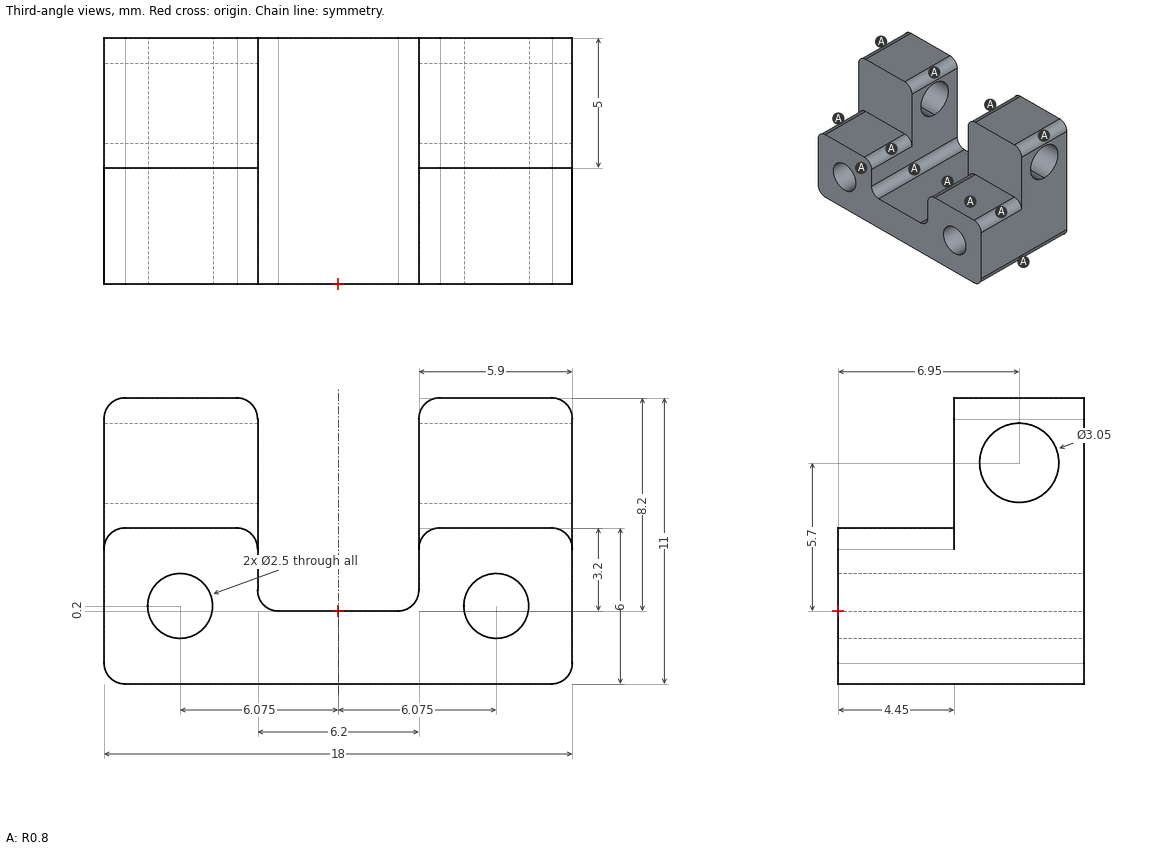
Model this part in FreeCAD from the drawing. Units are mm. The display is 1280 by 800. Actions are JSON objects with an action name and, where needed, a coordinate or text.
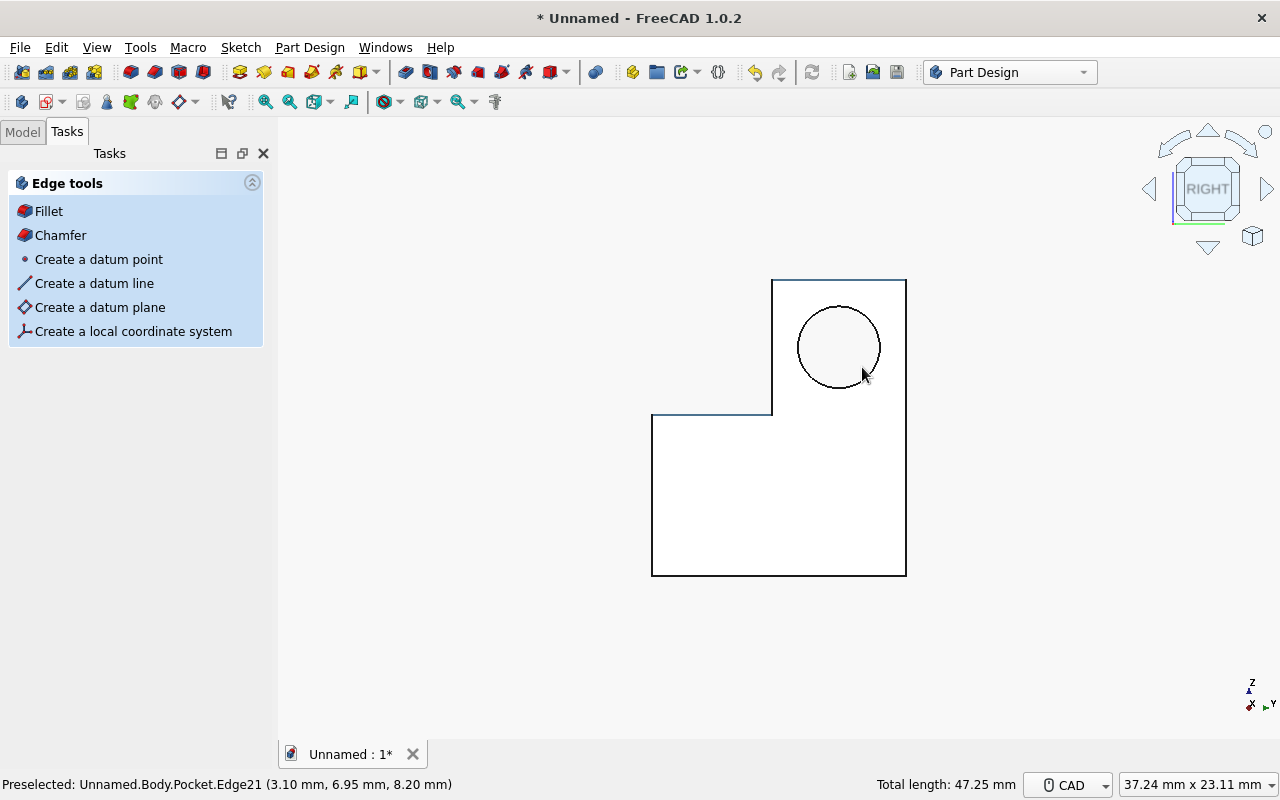
{"action": "left_click", "coordinate": [779, 575], "text": "ctrl"}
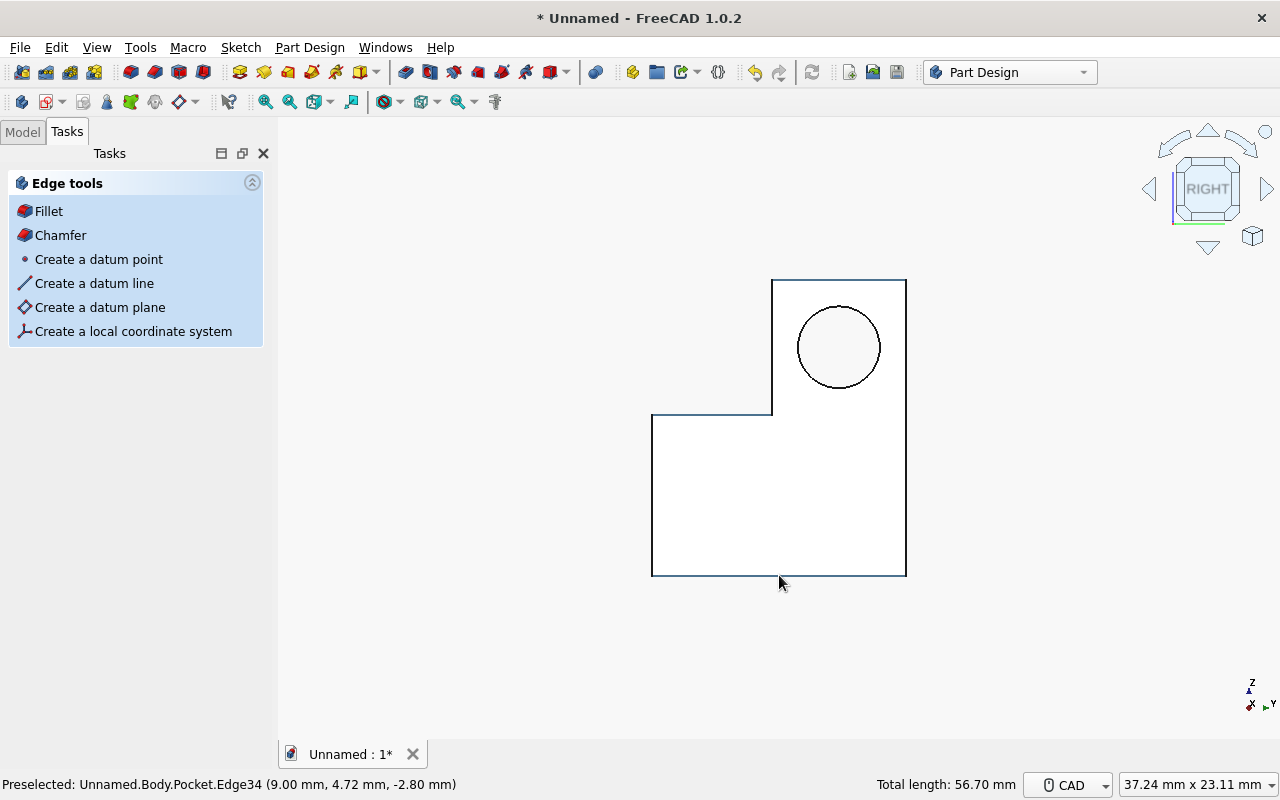
{"action": "key", "text": "5"}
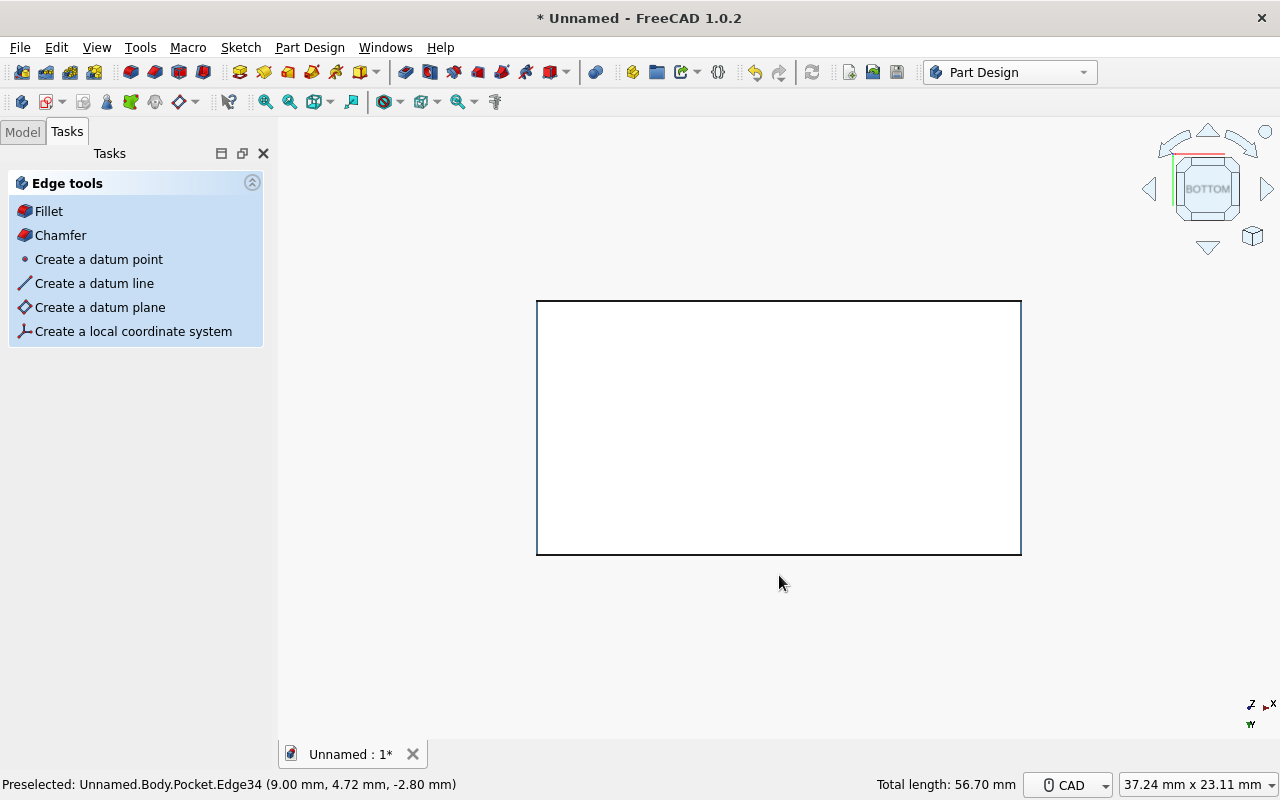
{"action": "key", "text": "4"}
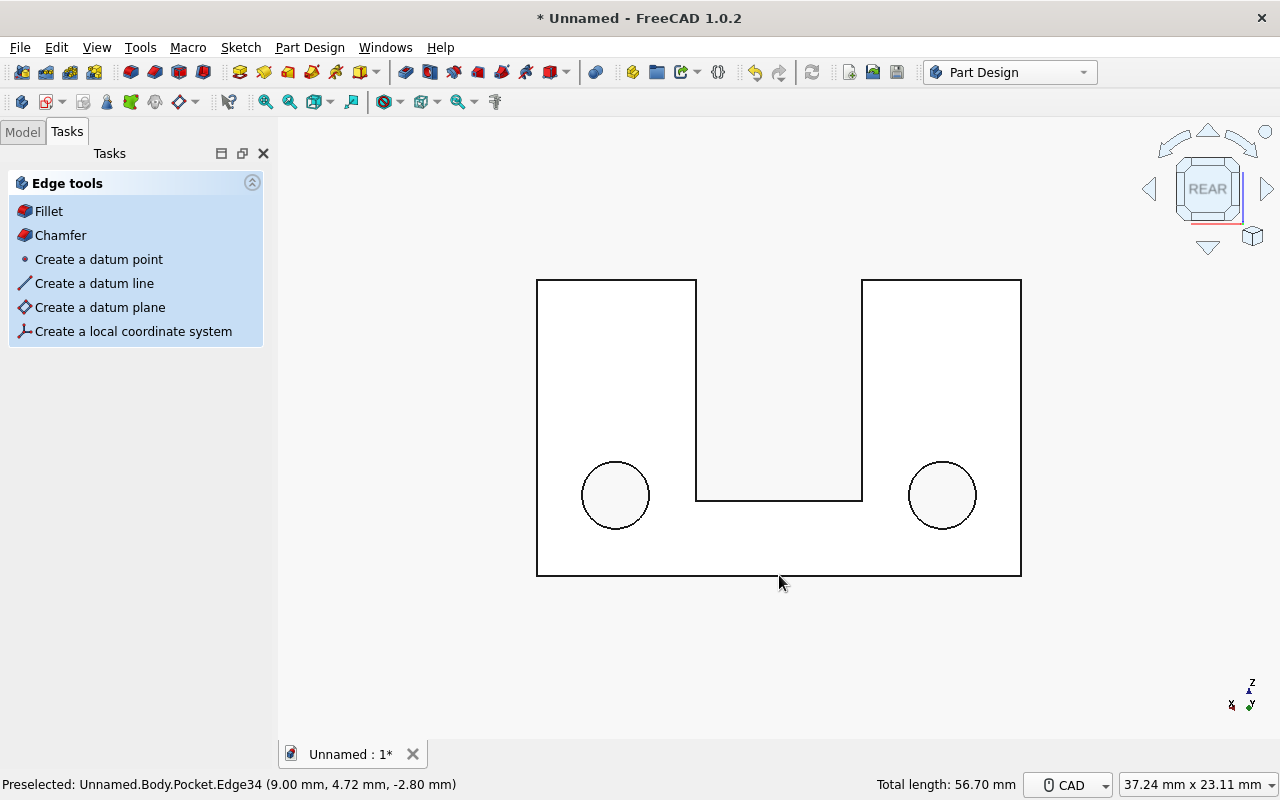
{"action": "key", "text": "6"}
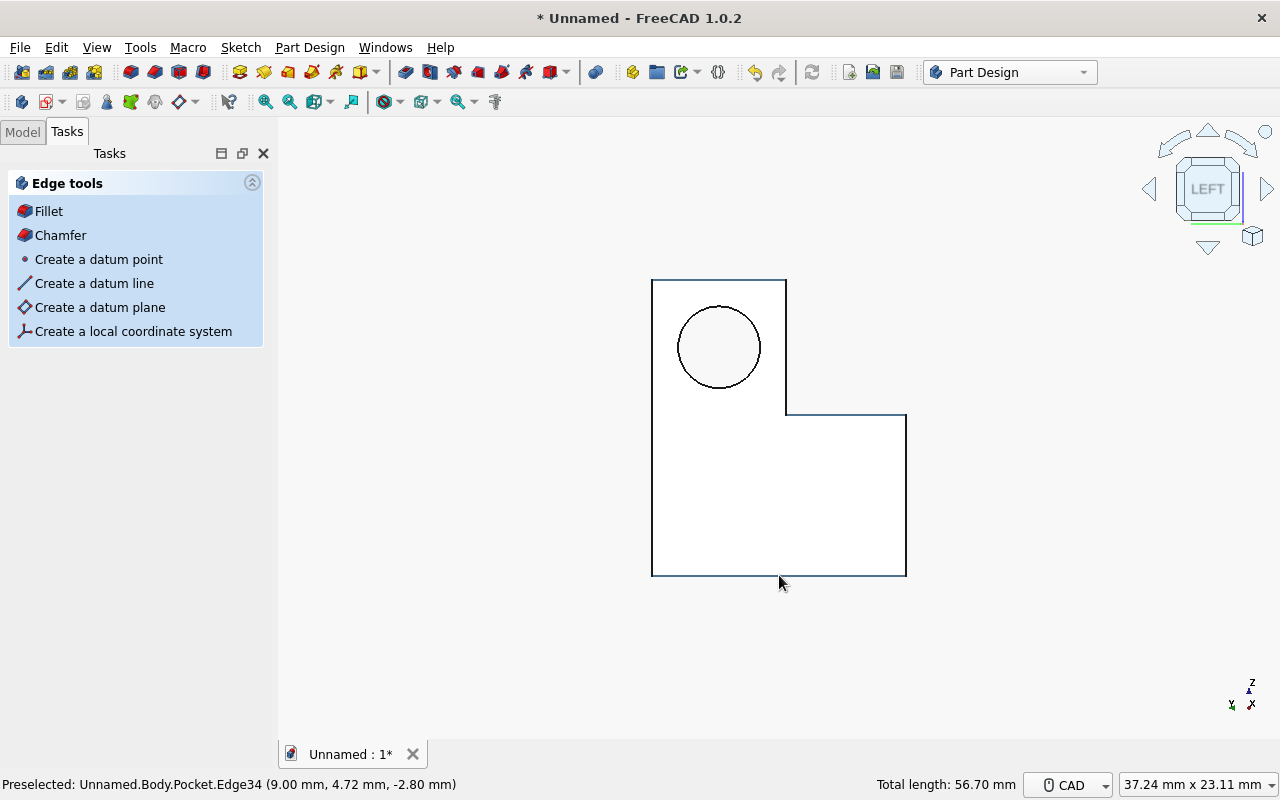
{"action": "key", "text": "v 3"}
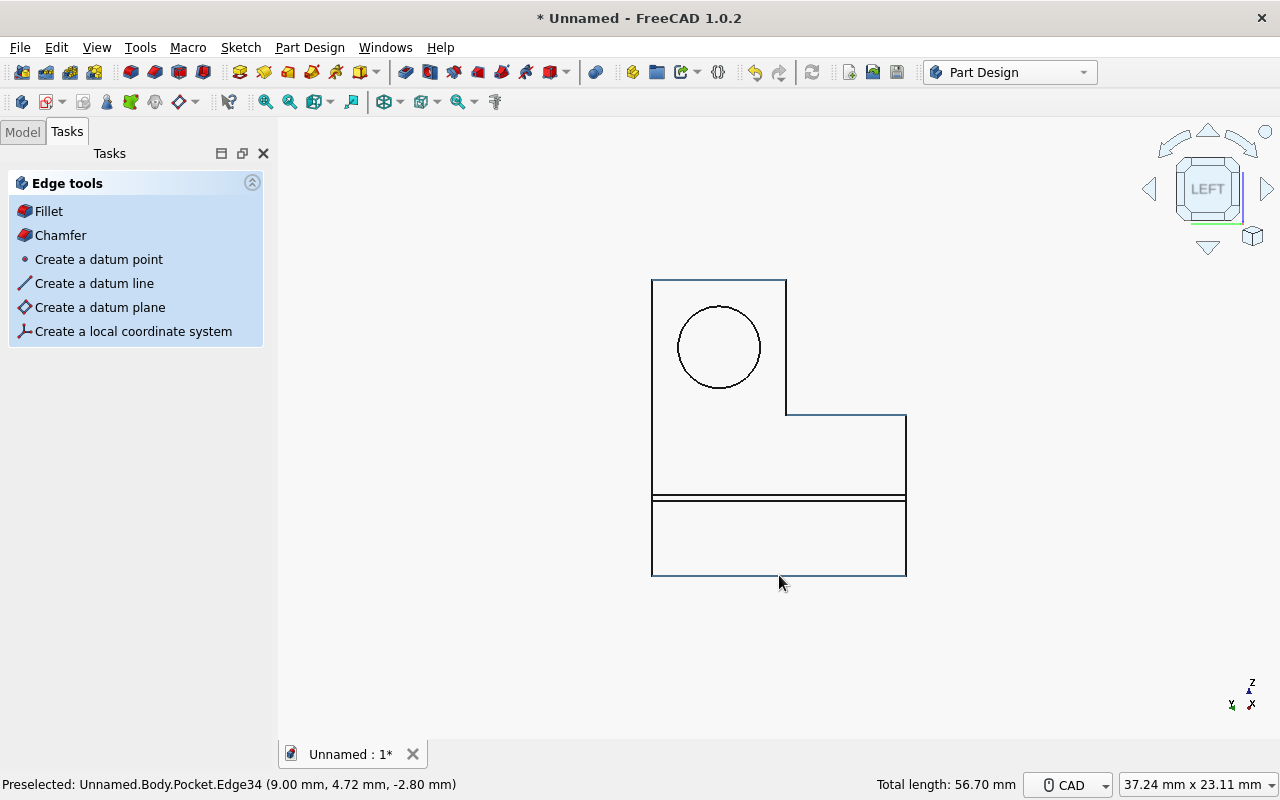
{"action": "key", "text": "0"}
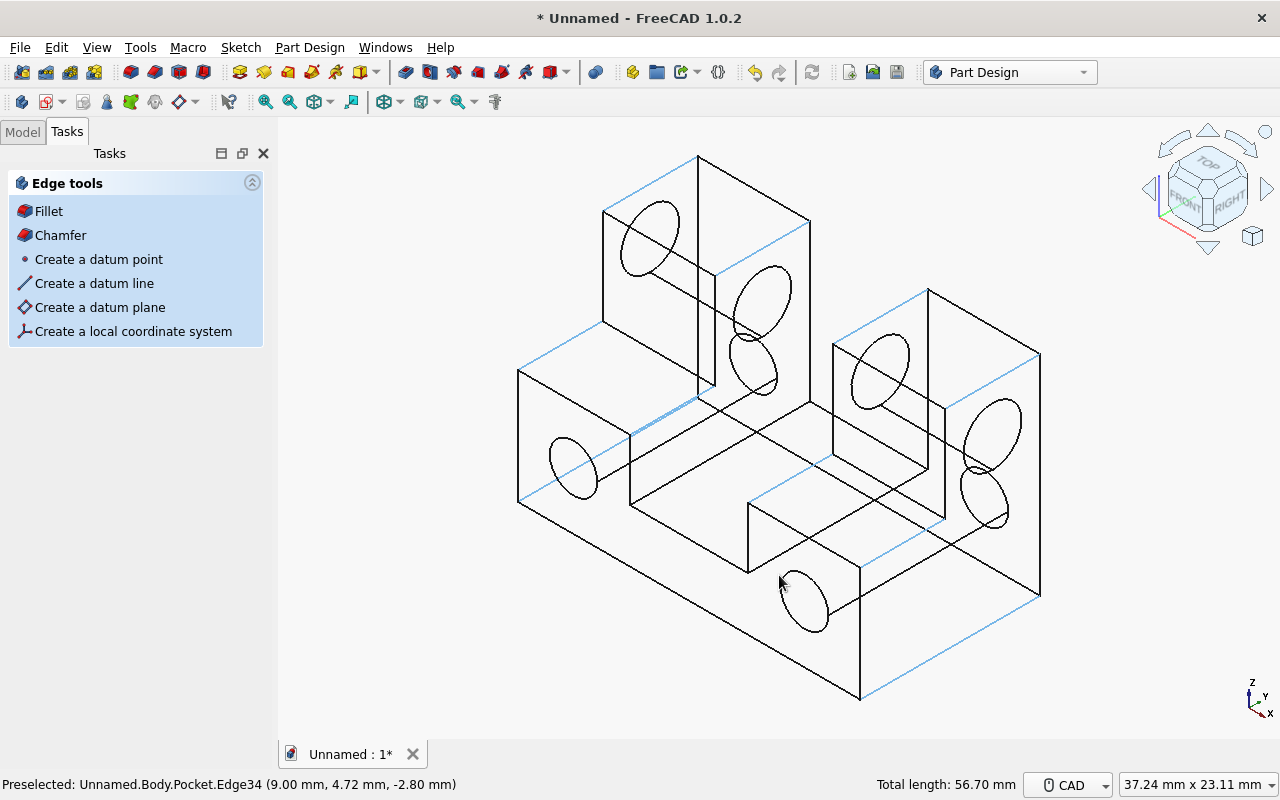
{"action": "left_click", "coordinate": [838, 520], "text": "ctrl"}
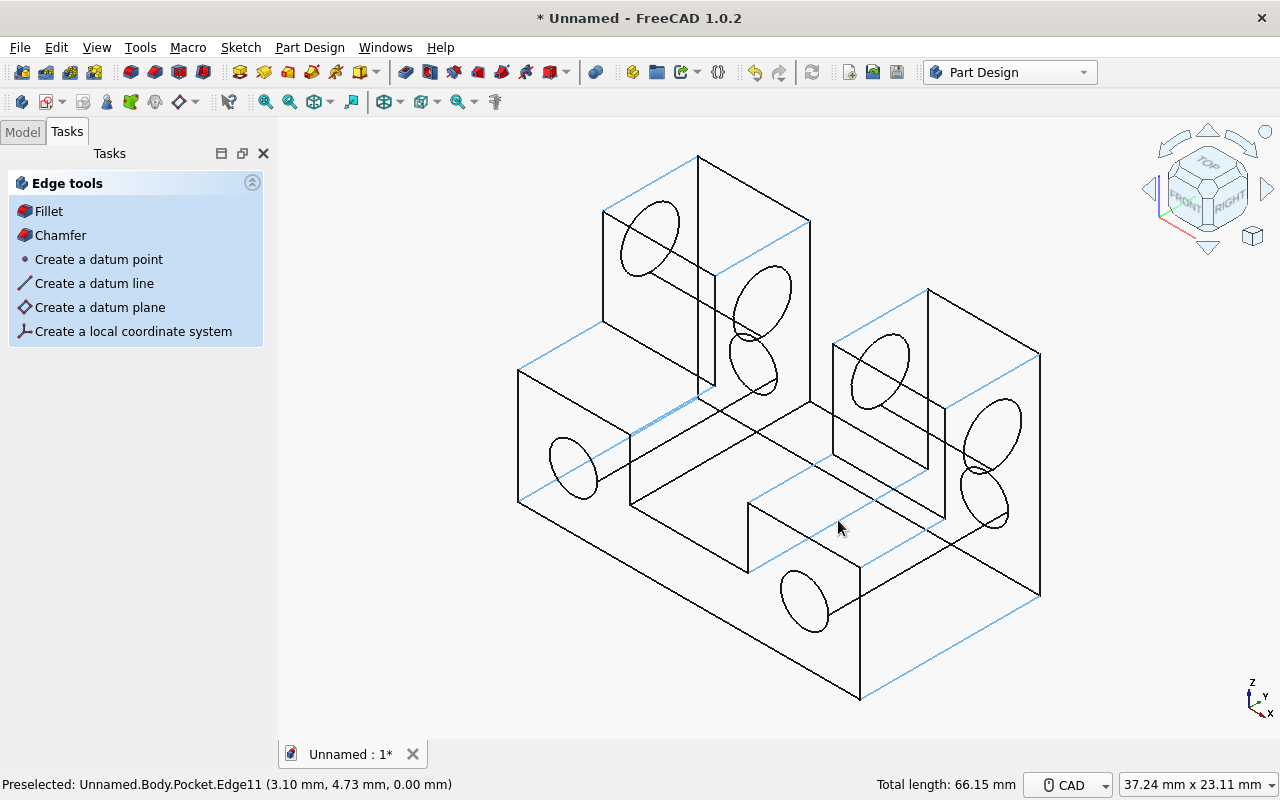
{"action": "left_click", "coordinate": [720, 452], "text": "ctrl"}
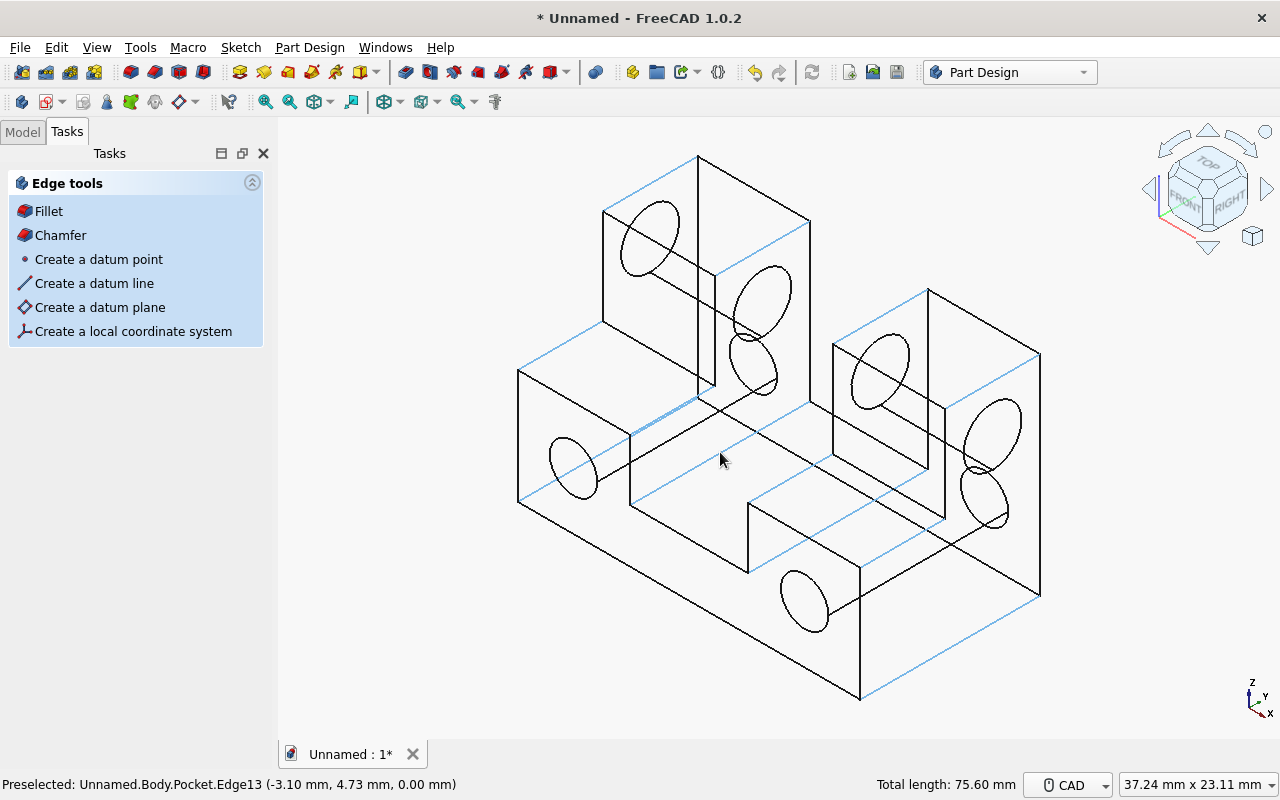
{"action": "key", "text": "v 1"}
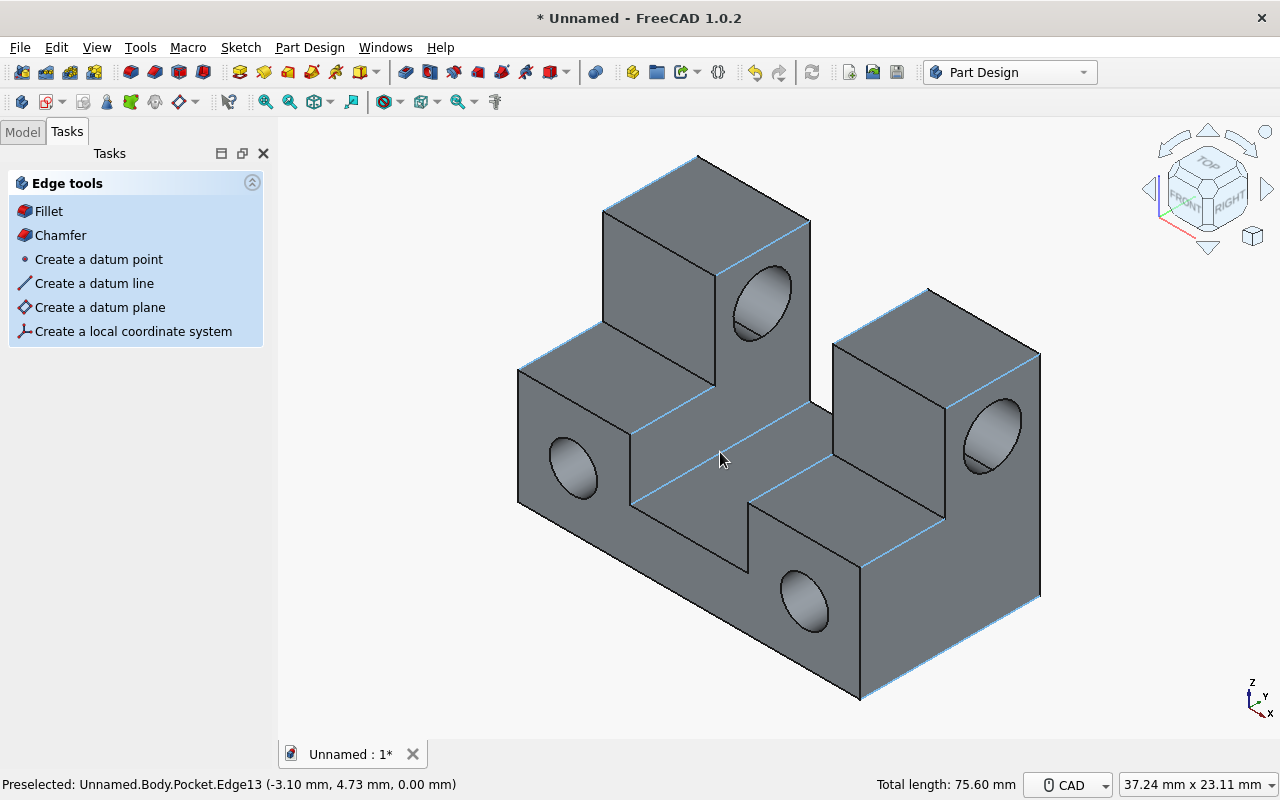
{"action": "left_click", "coordinate": [132, 72]}